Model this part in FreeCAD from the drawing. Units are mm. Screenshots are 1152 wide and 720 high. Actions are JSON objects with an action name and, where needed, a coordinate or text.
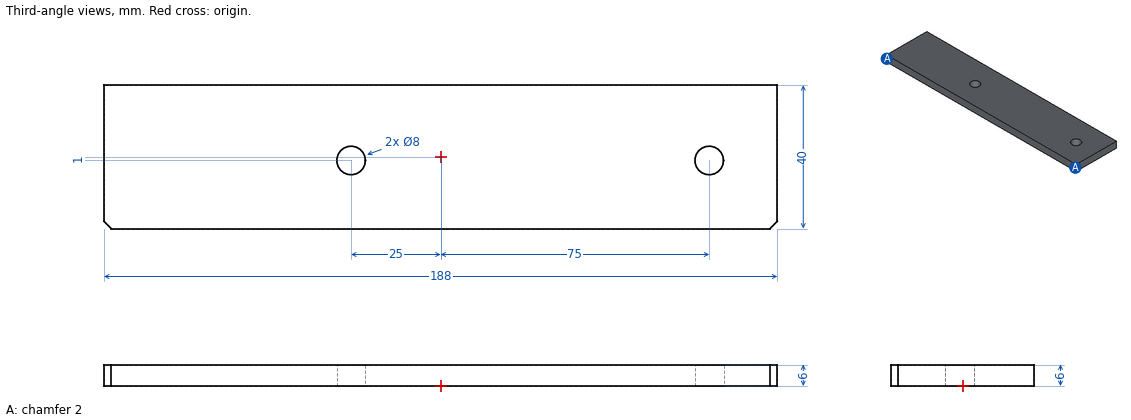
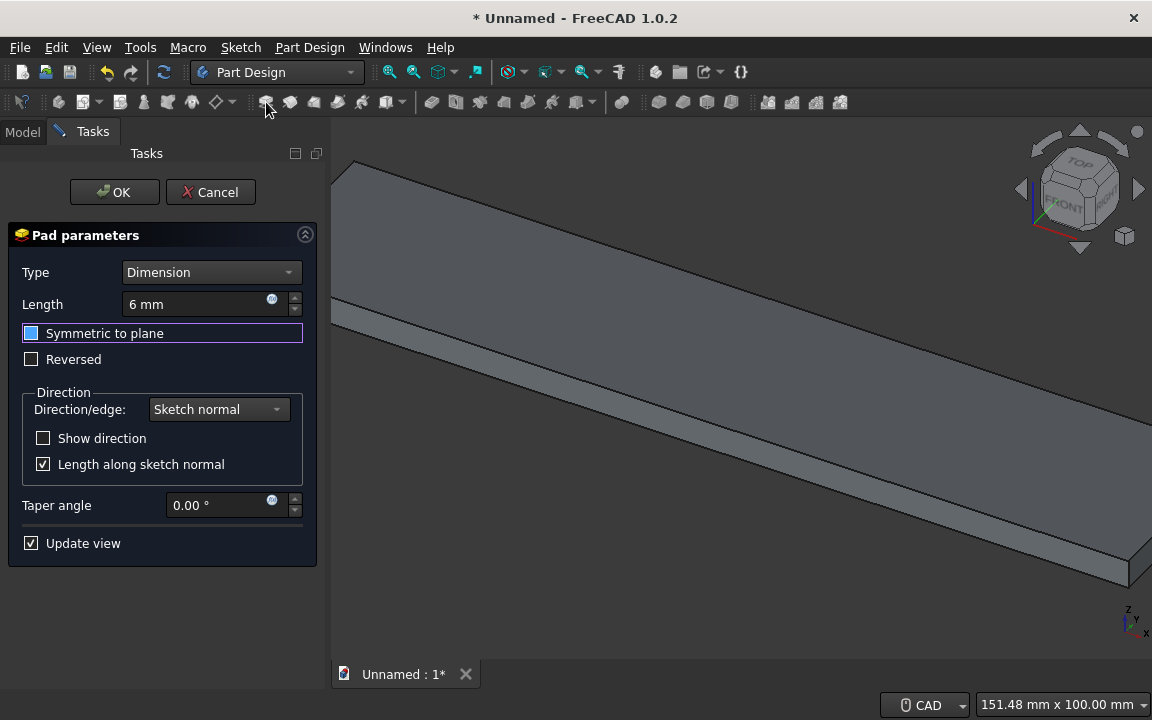
{"action": "left_click", "coordinate": [115, 192]}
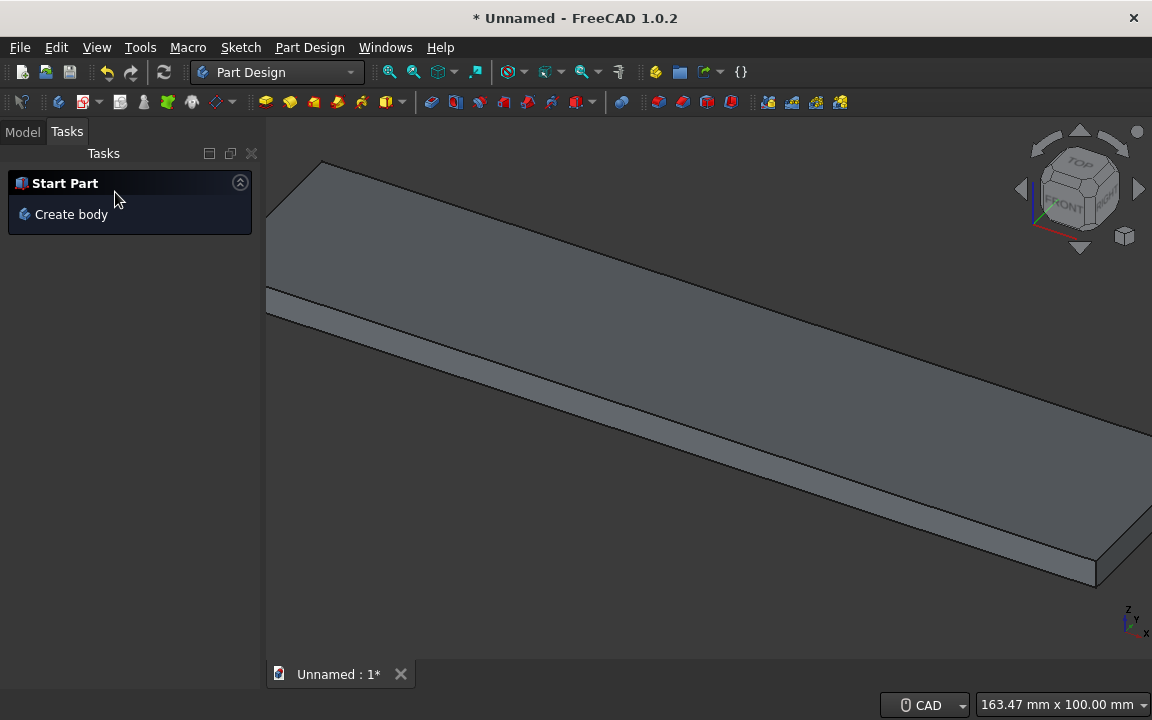
{"action": "left_click", "coordinate": [390, 72]}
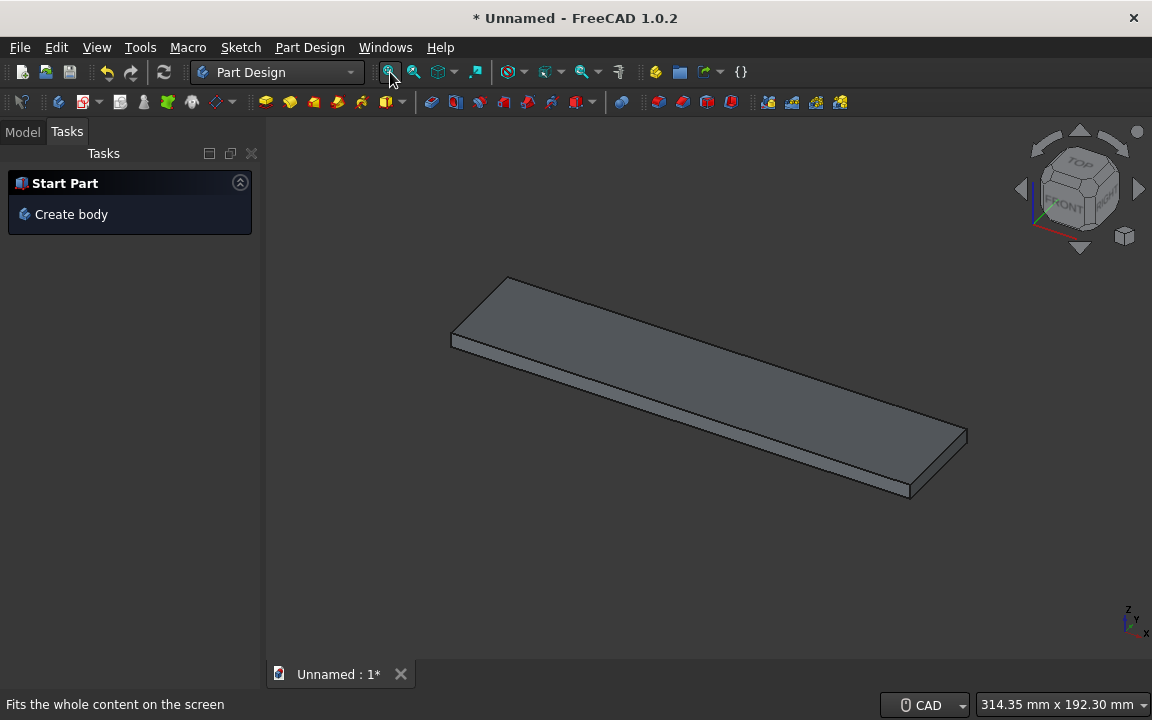
{"action": "left_click", "coordinate": [840, 423]}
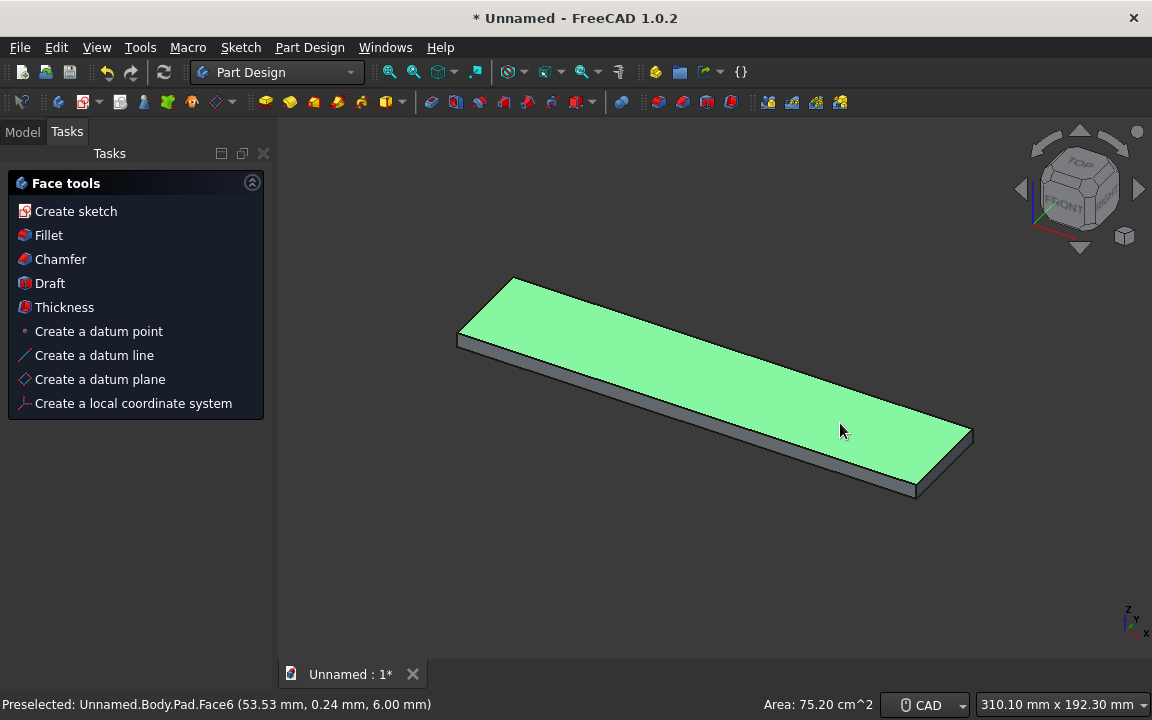
{"action": "left_click", "coordinate": [84, 102]}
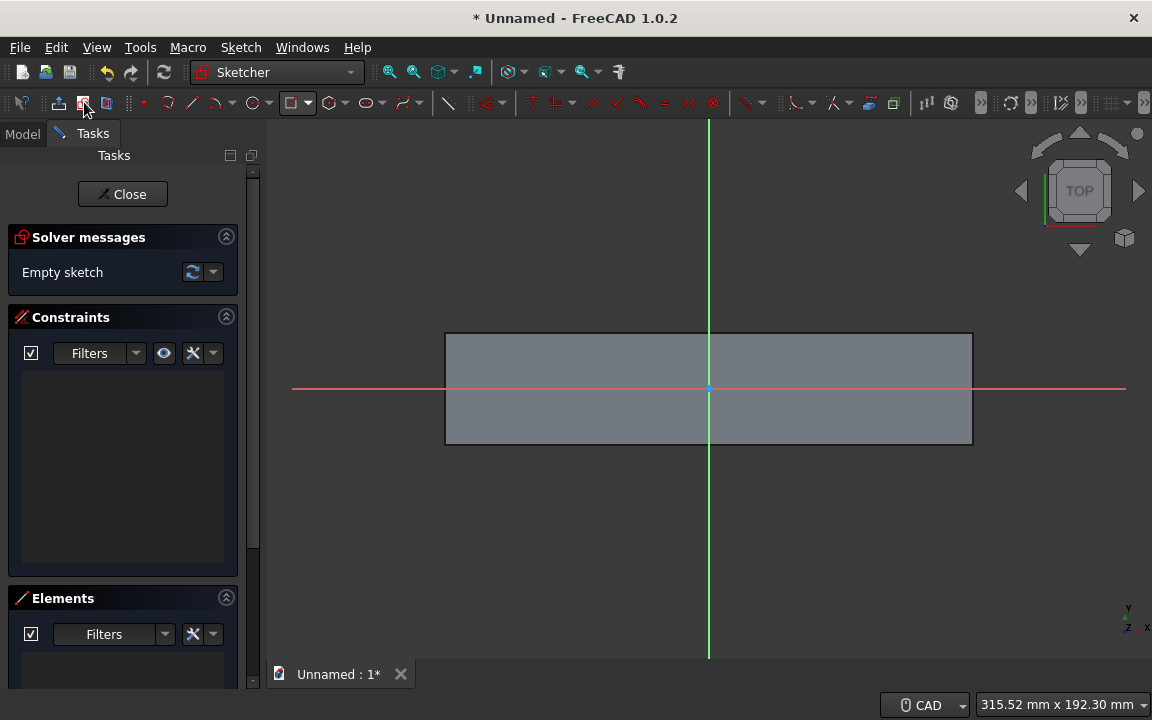
{"action": "scroll", "coordinate": [987, 398], "scroll_direction": "up", "scroll_amount": 2}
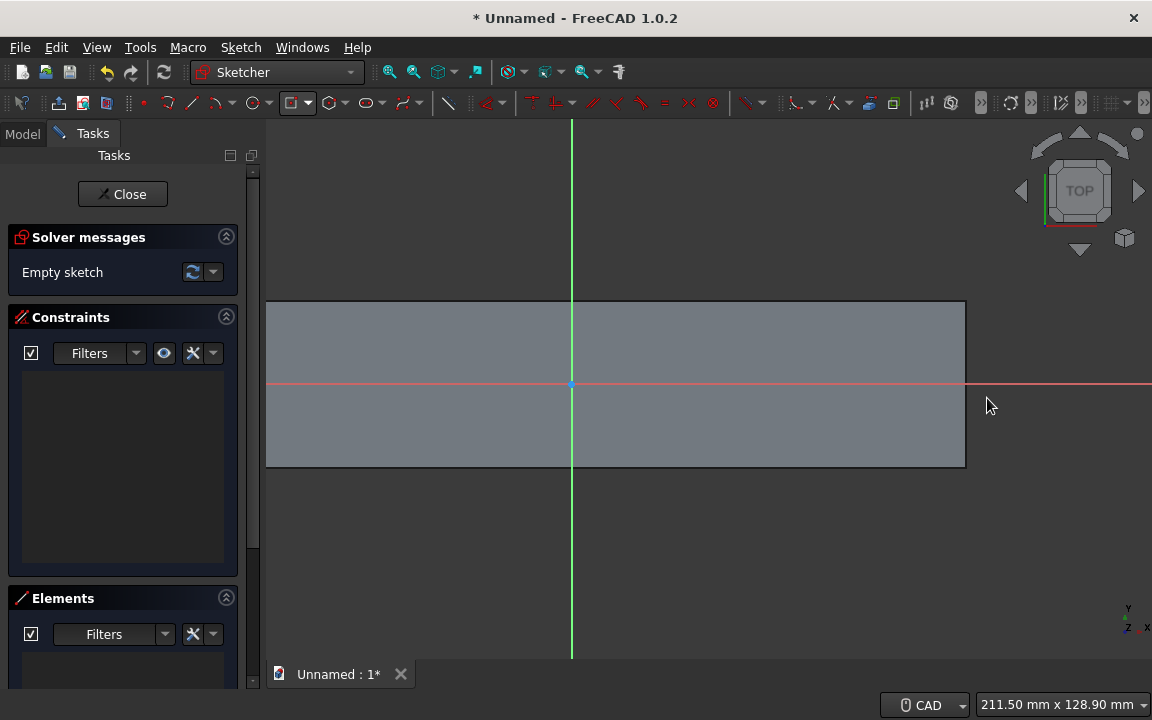
{"action": "left_click", "coordinate": [254, 104]}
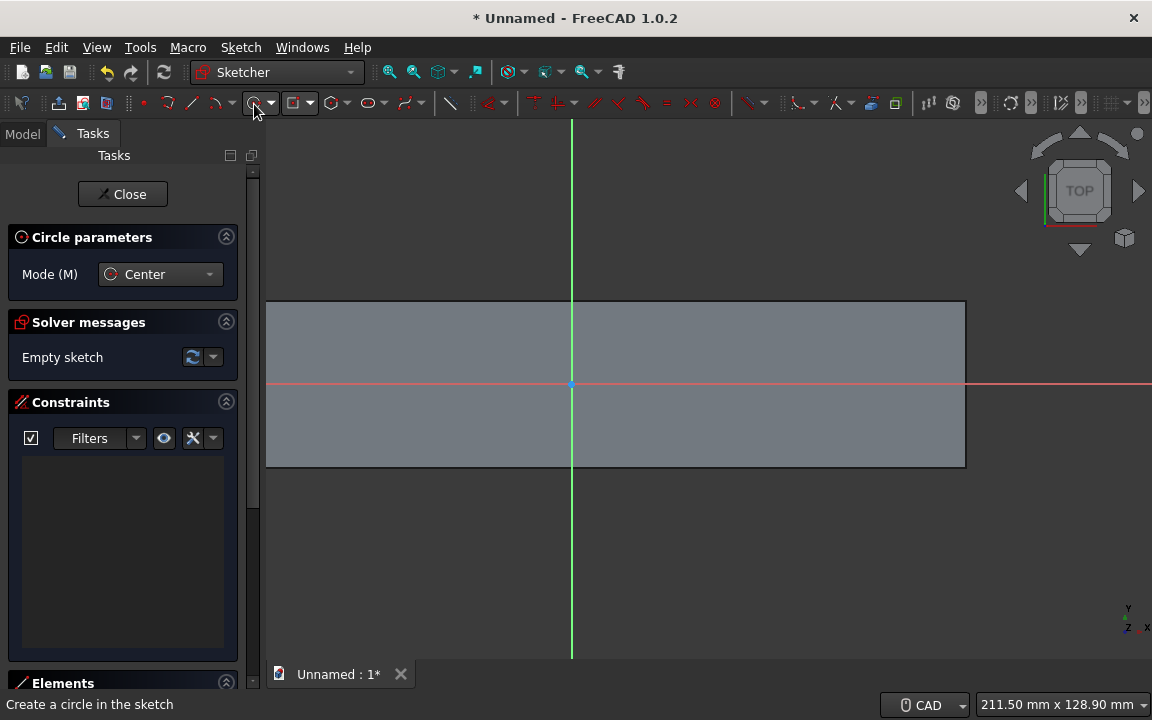
{"action": "scroll", "coordinate": [467, 389], "scroll_direction": "up", "scroll_amount": 7}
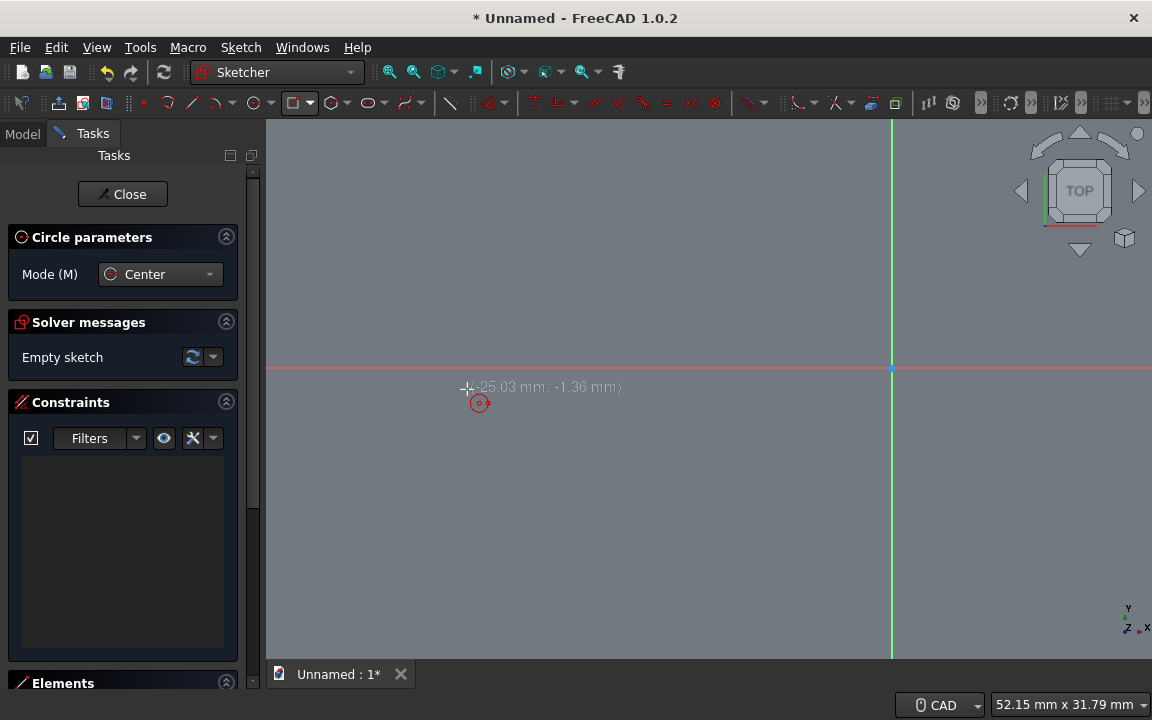
{"action": "left_click", "coordinate": [467, 385]}
{"action": "mouse_move", "coordinate": [515, 337]}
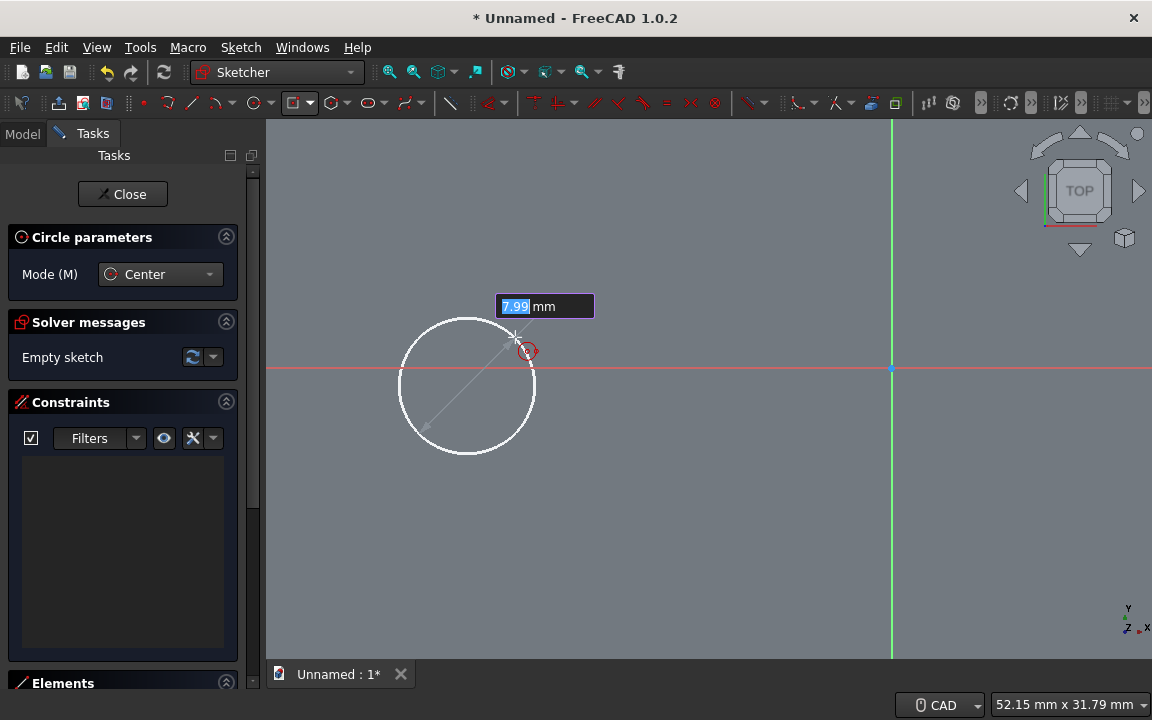
{"action": "type", "text": "8"}
{"action": "key", "text": "Return"}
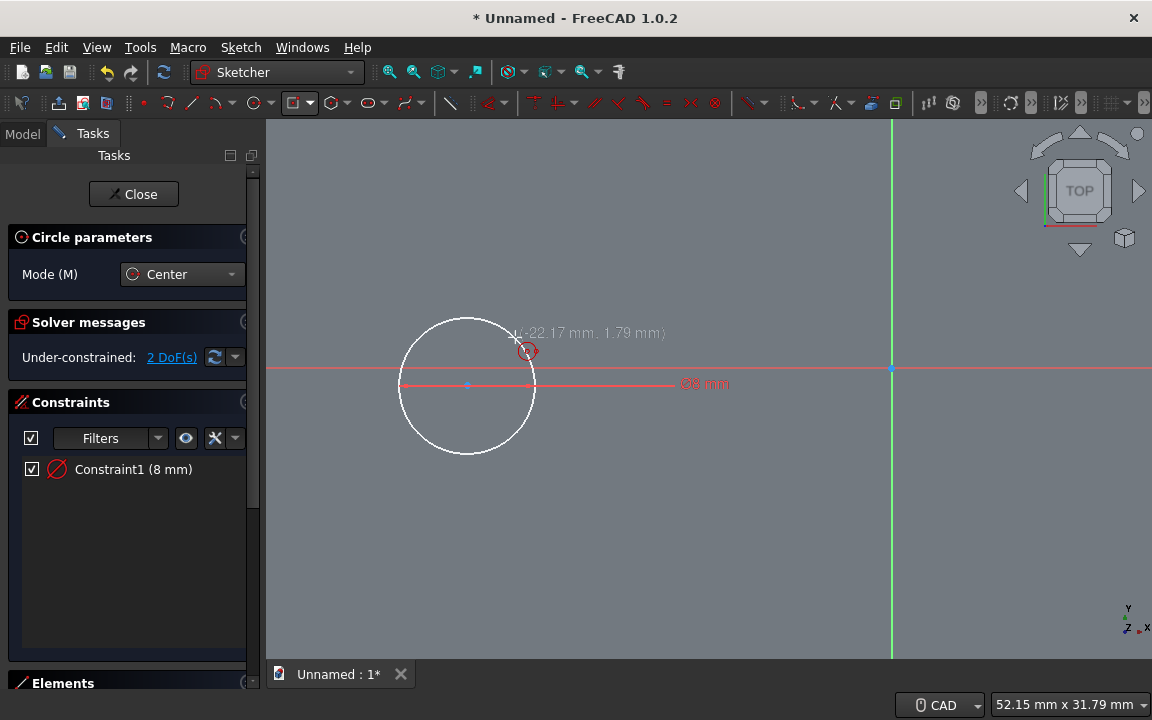
{"action": "scroll", "coordinate": [419, 390], "scroll_direction": "down", "scroll_amount": 7}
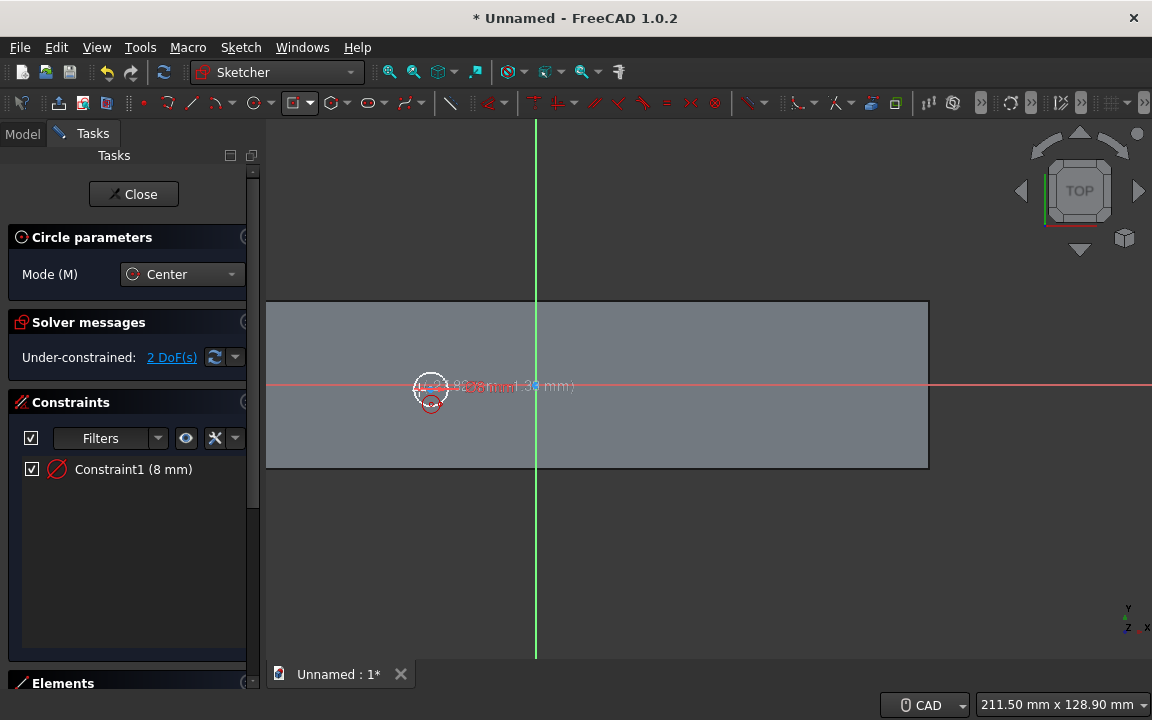
{"action": "scroll", "coordinate": [850, 389], "scroll_direction": "up", "scroll_amount": 7}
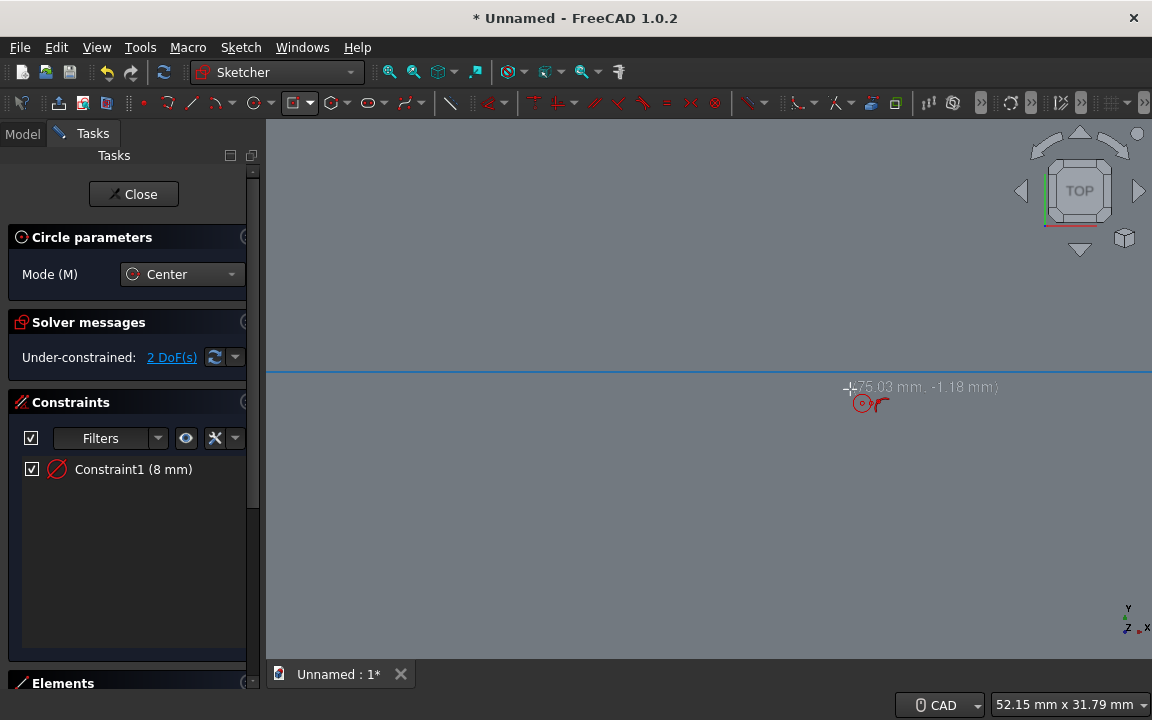
{"action": "left_click", "coordinate": [847, 389]}
{"action": "mouse_move", "coordinate": [895, 340]}